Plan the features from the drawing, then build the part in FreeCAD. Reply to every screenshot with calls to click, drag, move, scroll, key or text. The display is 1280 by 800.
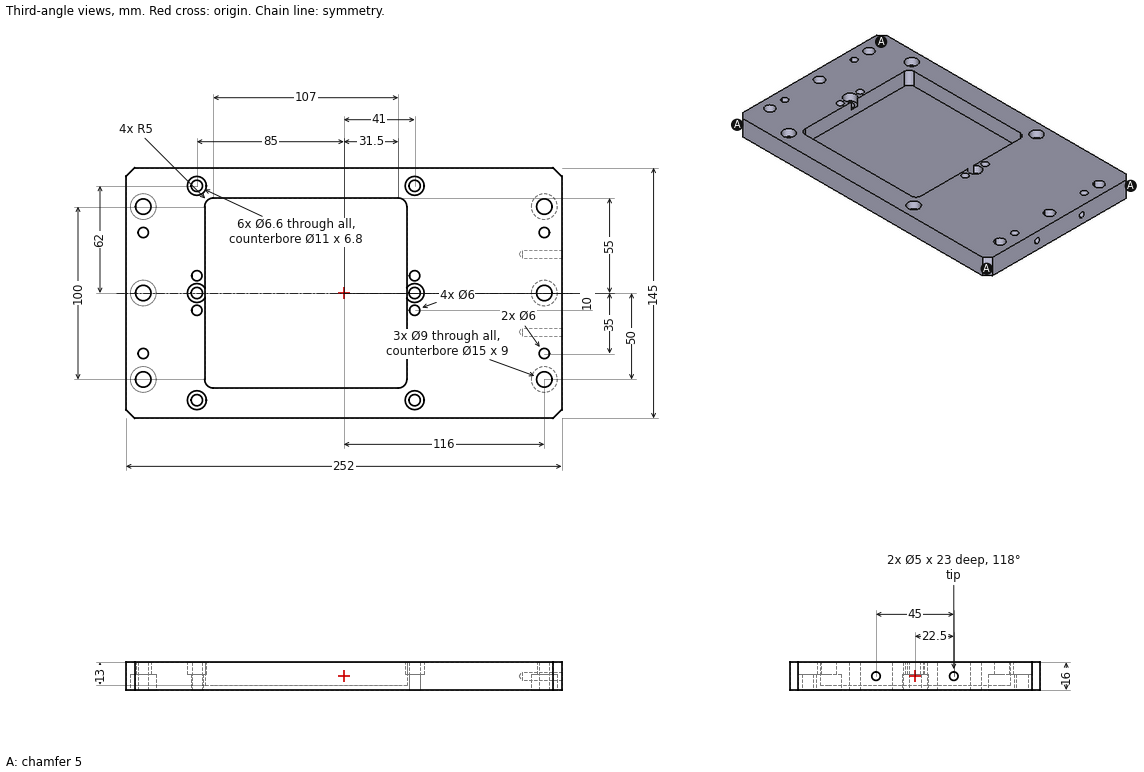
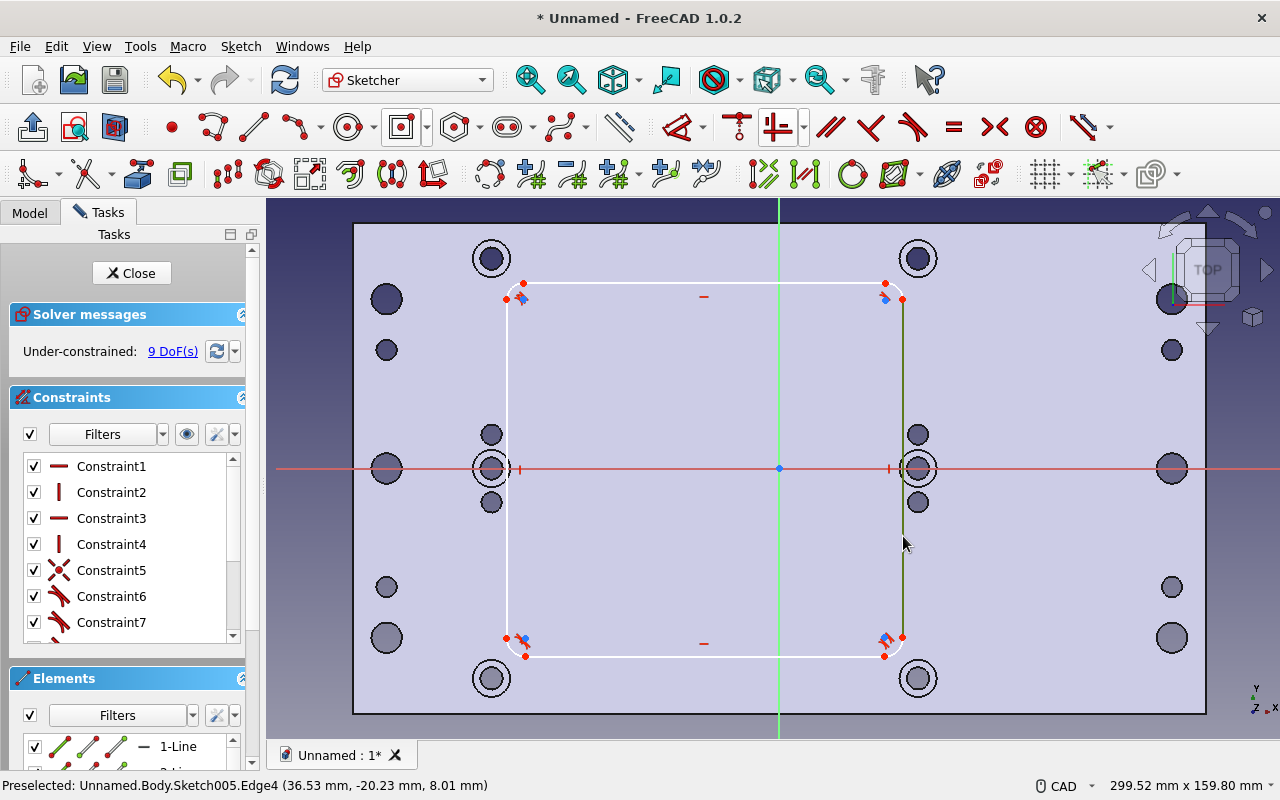
click(898, 288)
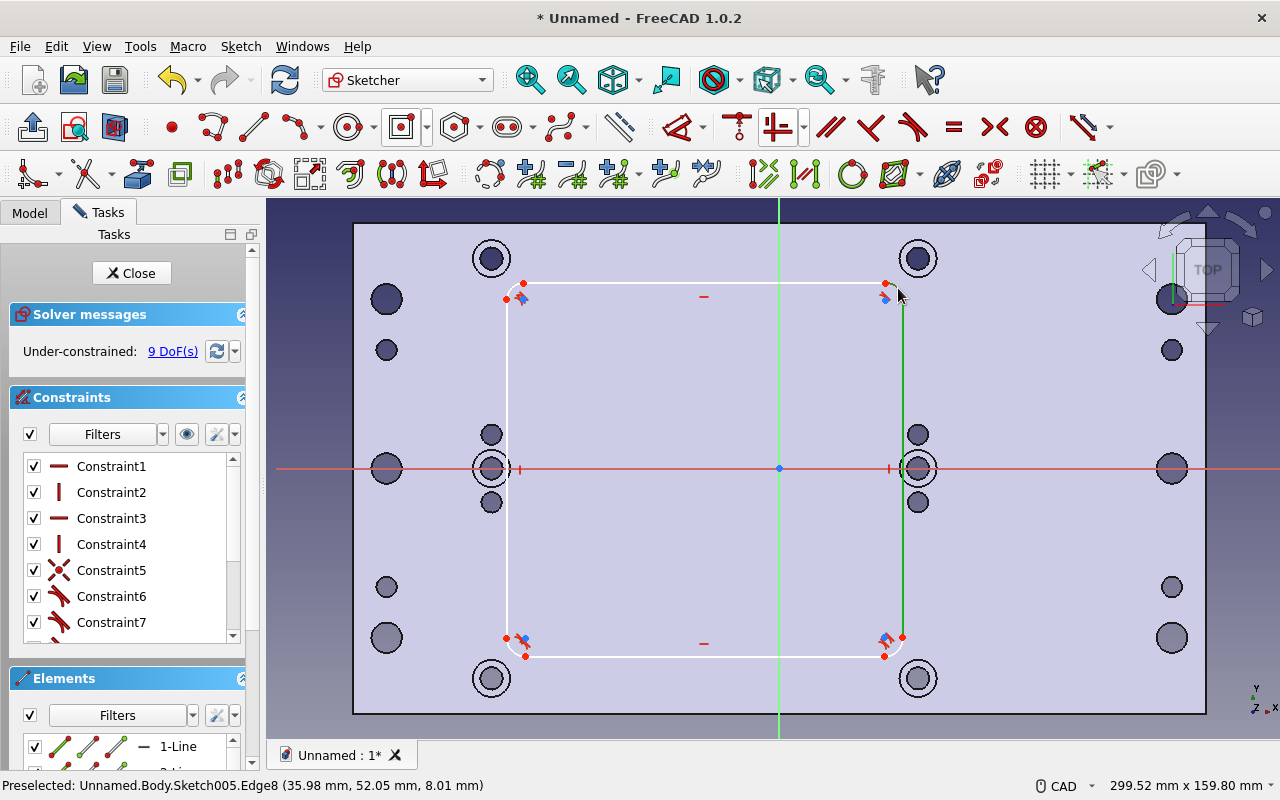
key(t)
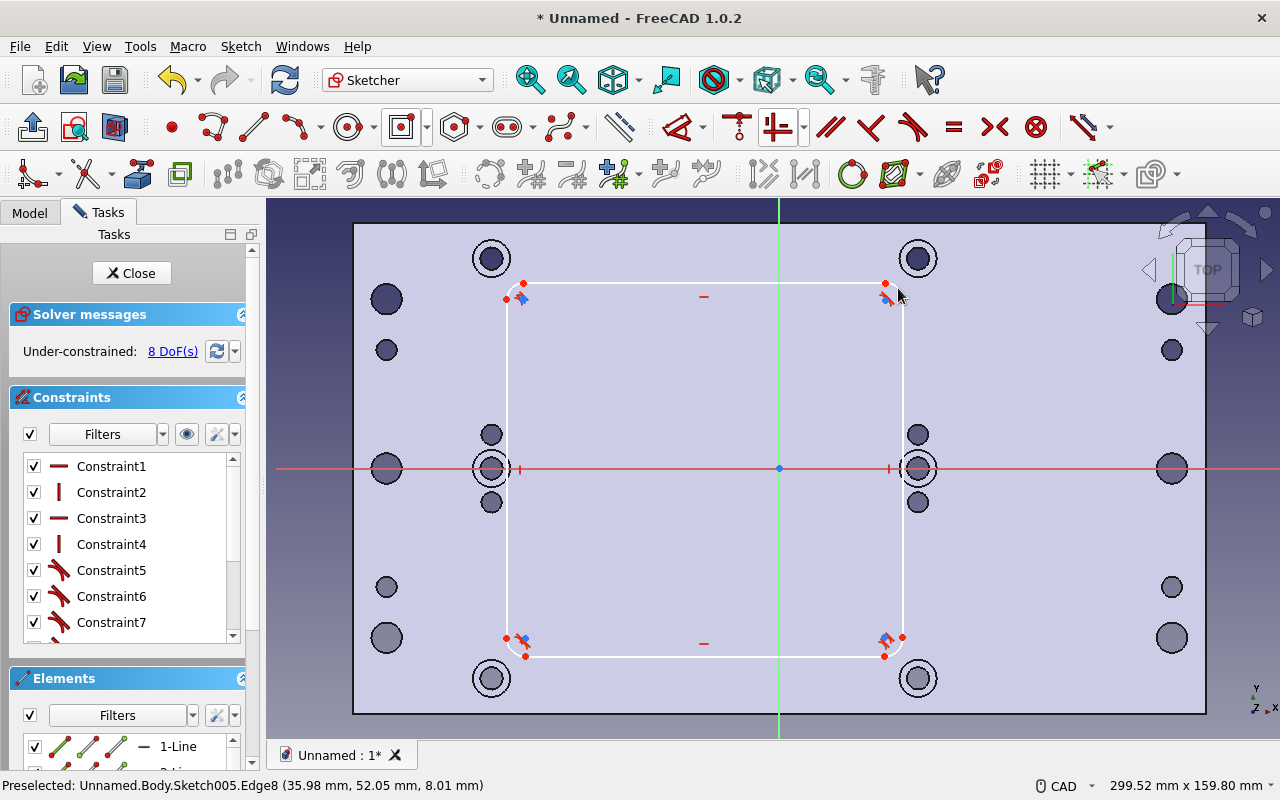
click(512, 288)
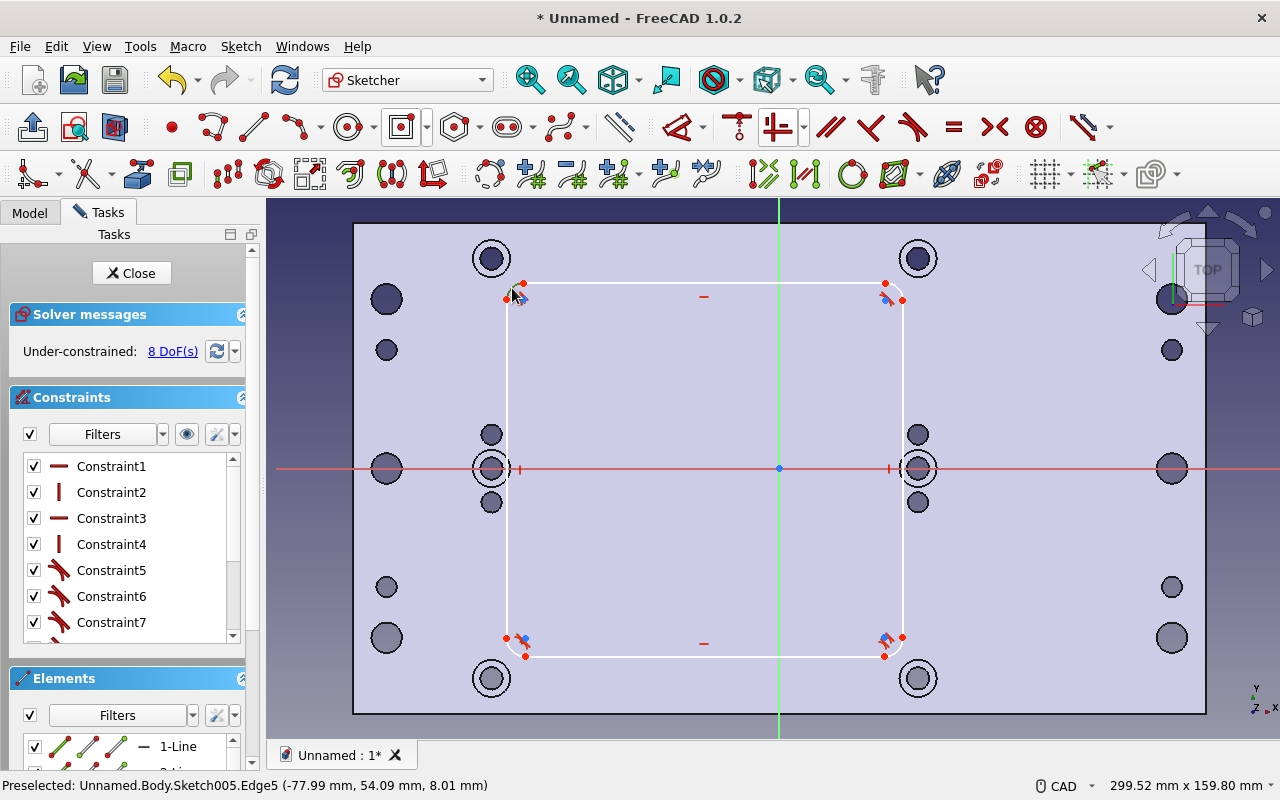
click(512, 651)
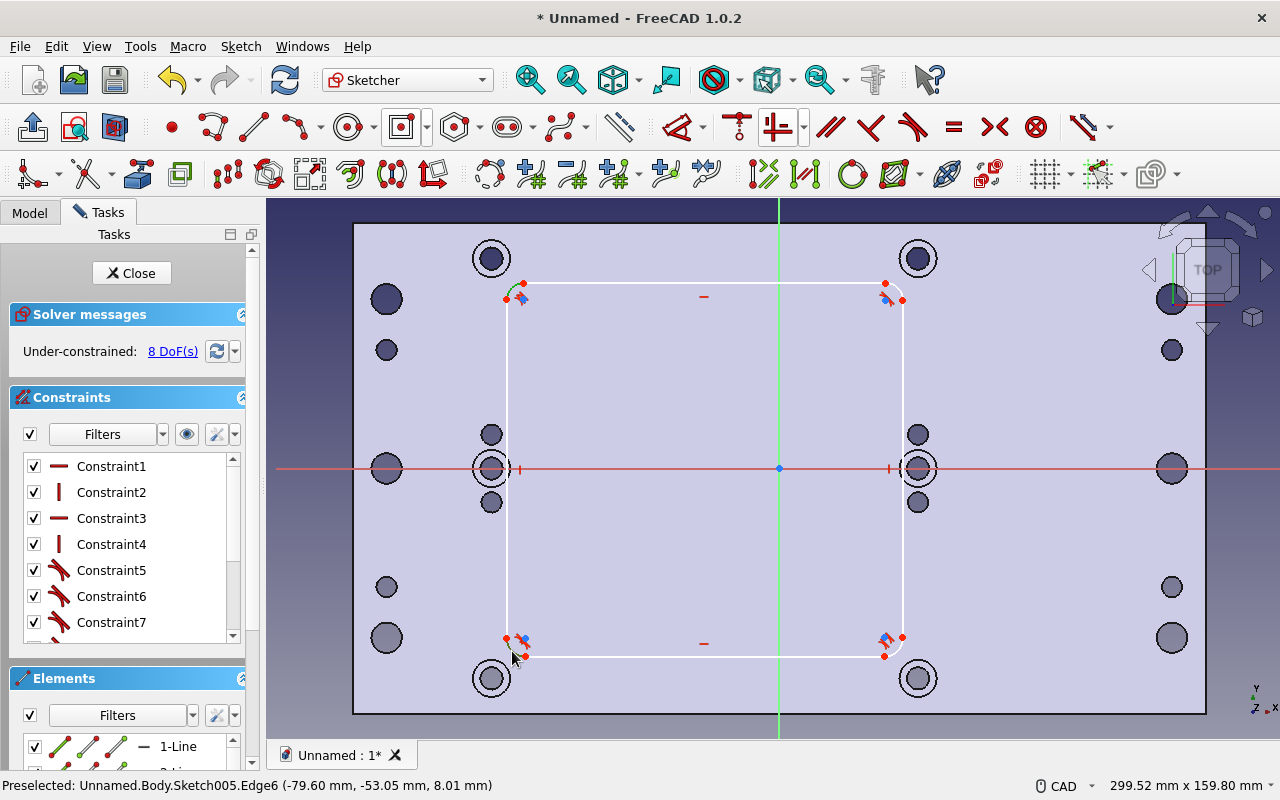
click(897, 651)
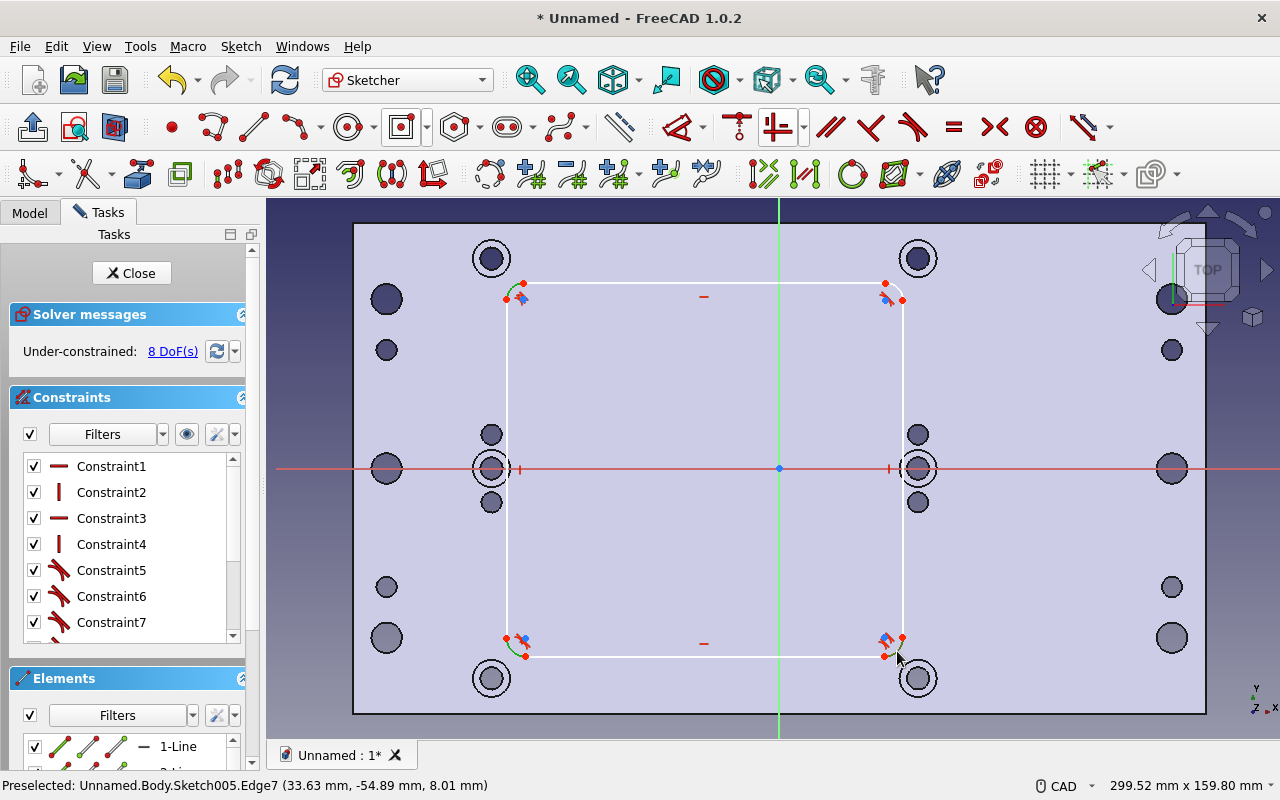
click(898, 288)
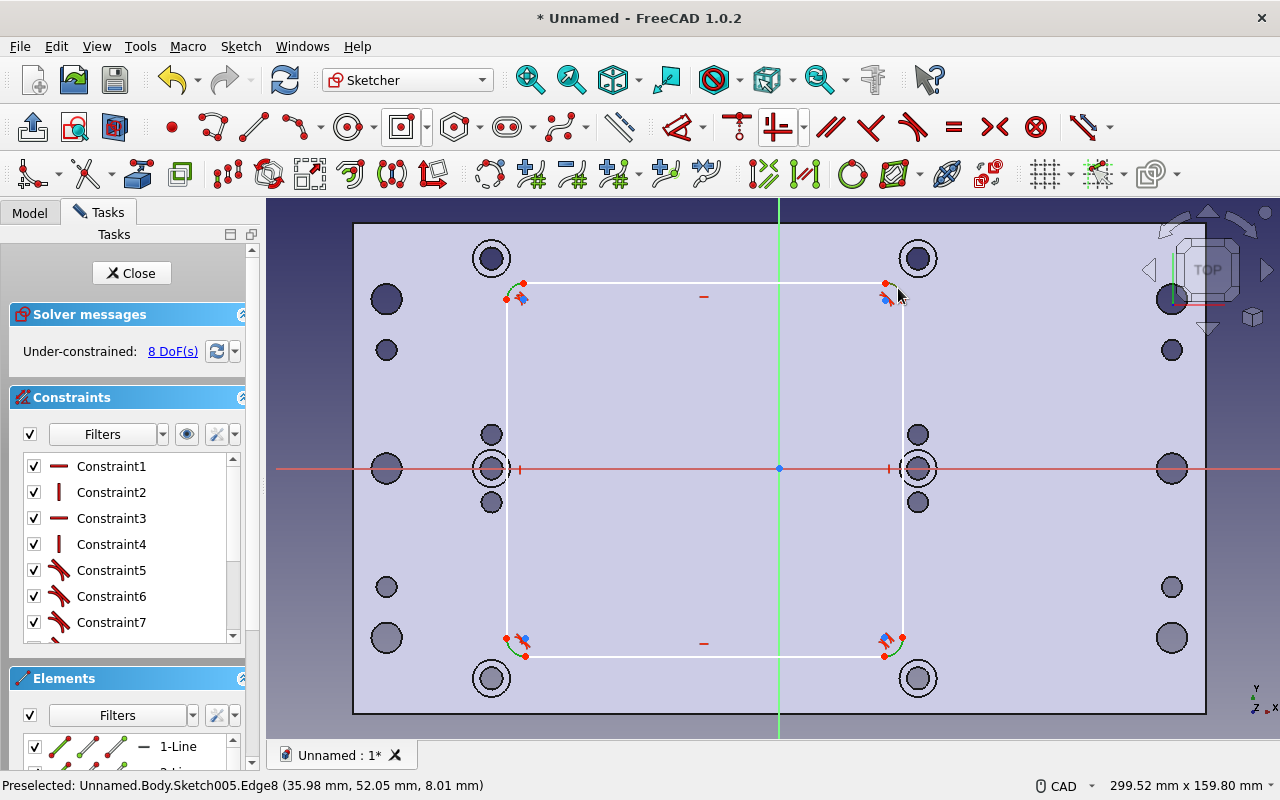
key(e)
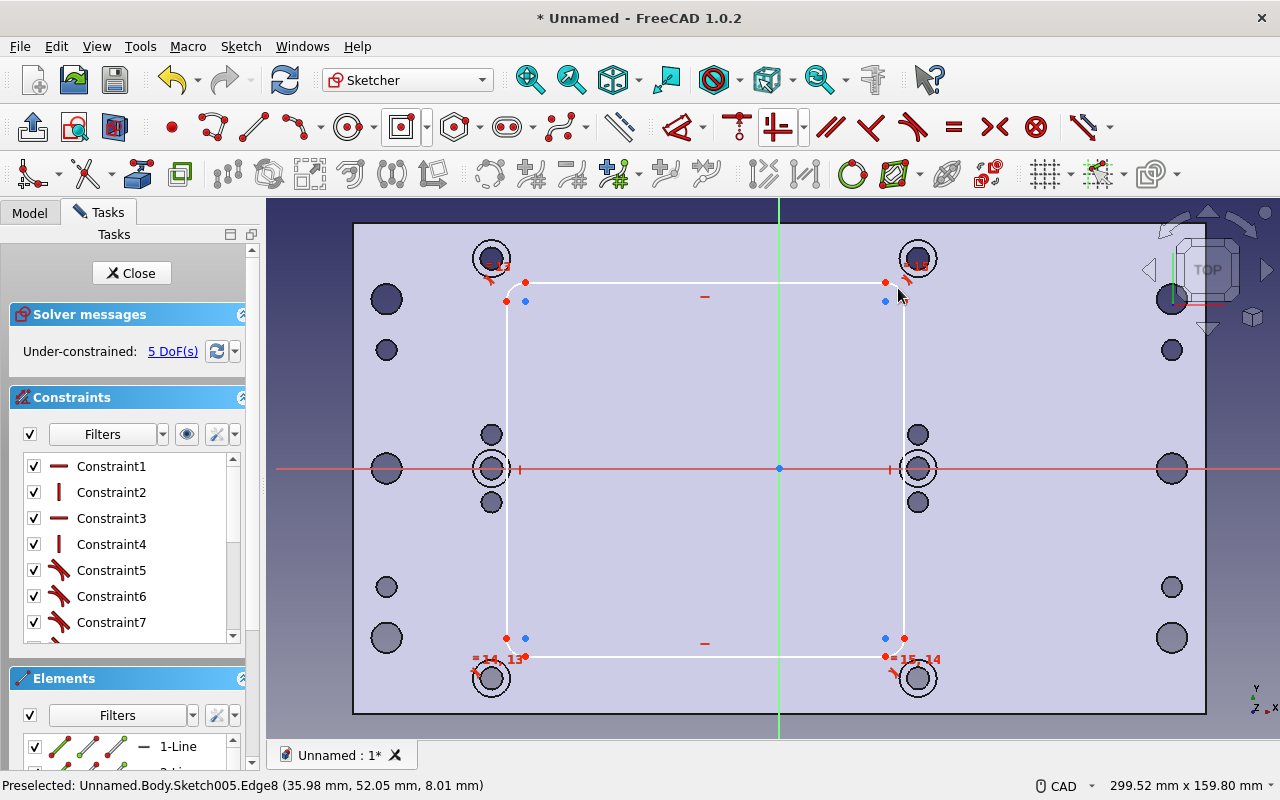
key(d)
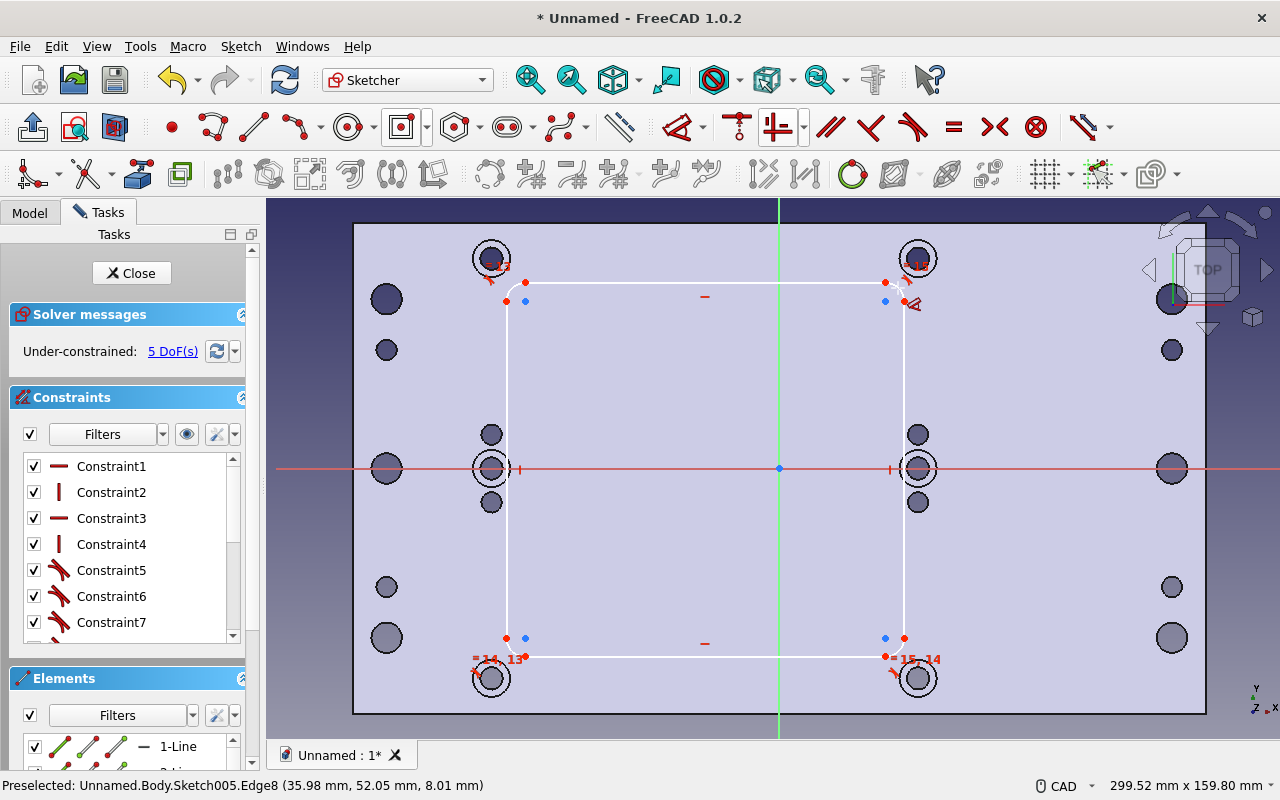
scroll(512, 288, up, 5)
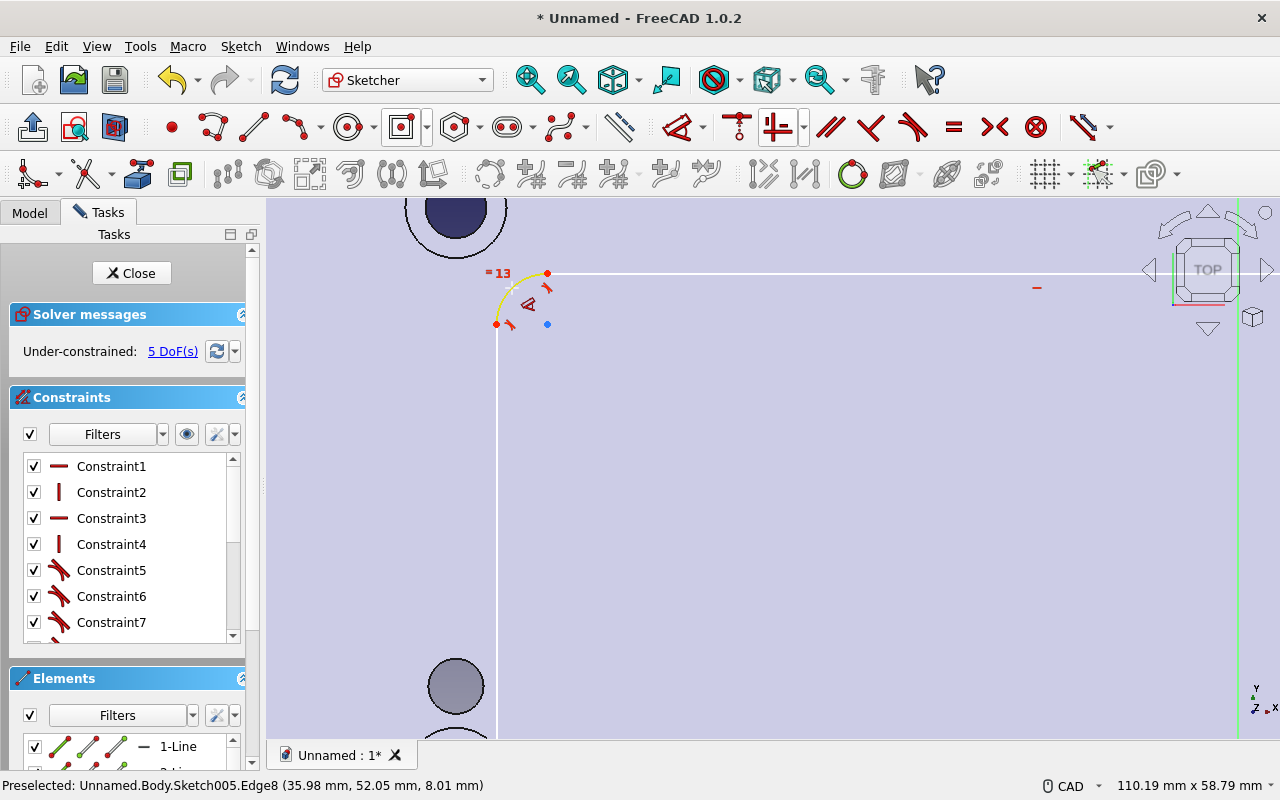
click(512, 289)
click(489, 266)